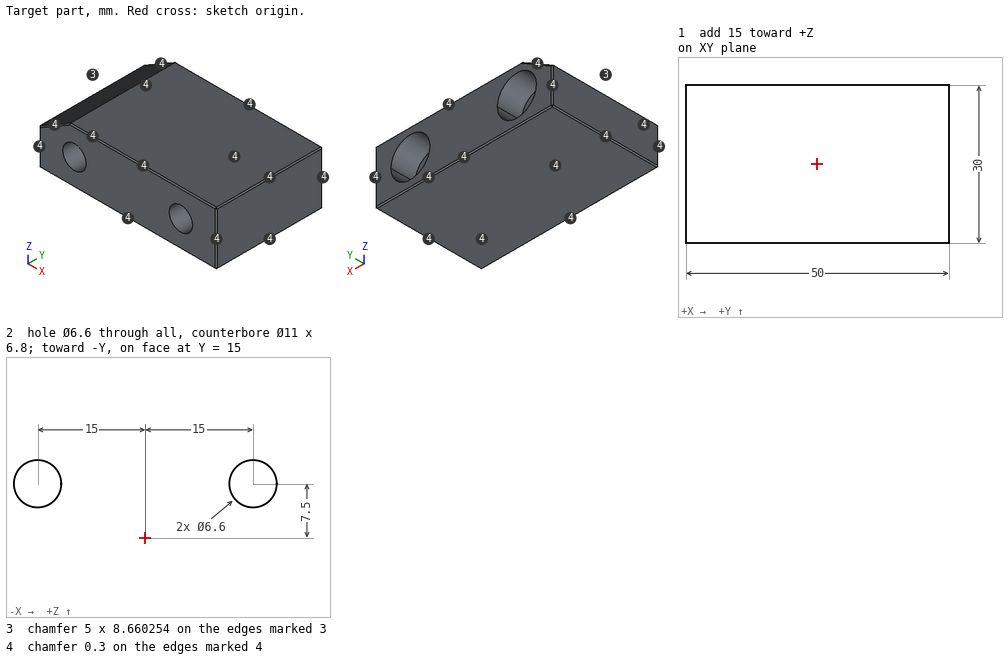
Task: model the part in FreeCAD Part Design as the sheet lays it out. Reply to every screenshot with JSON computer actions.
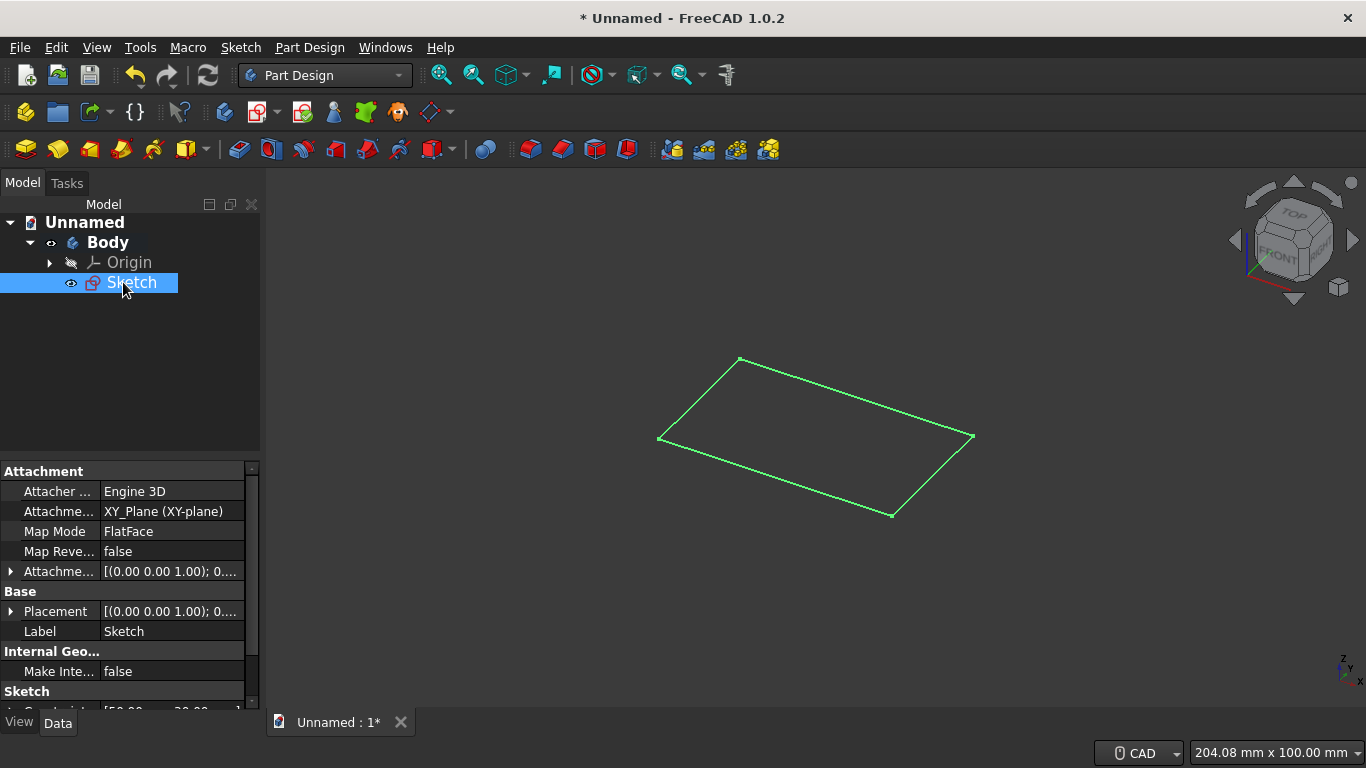
{"action": "left_click", "coordinate": [26, 150]}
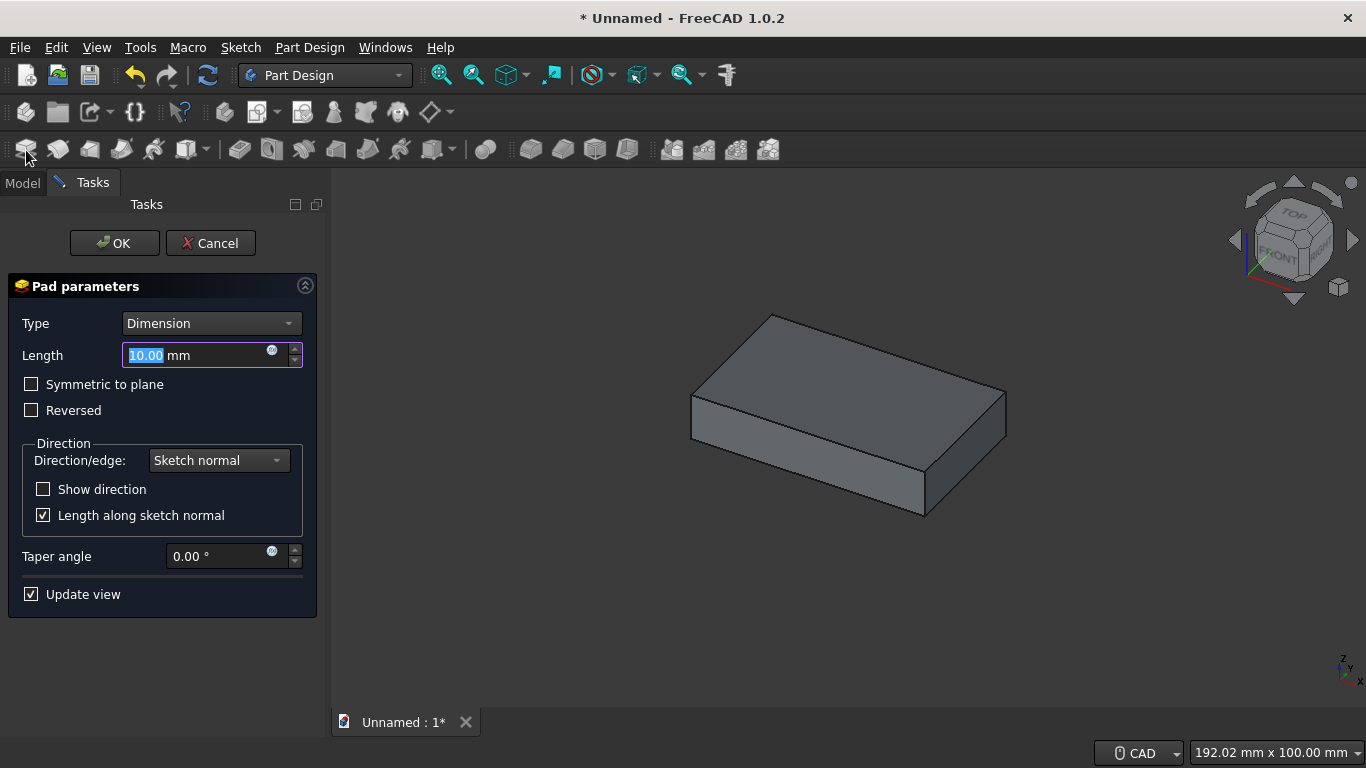
{"action": "type", "text": "15"}
{"action": "key", "text": "Tab"}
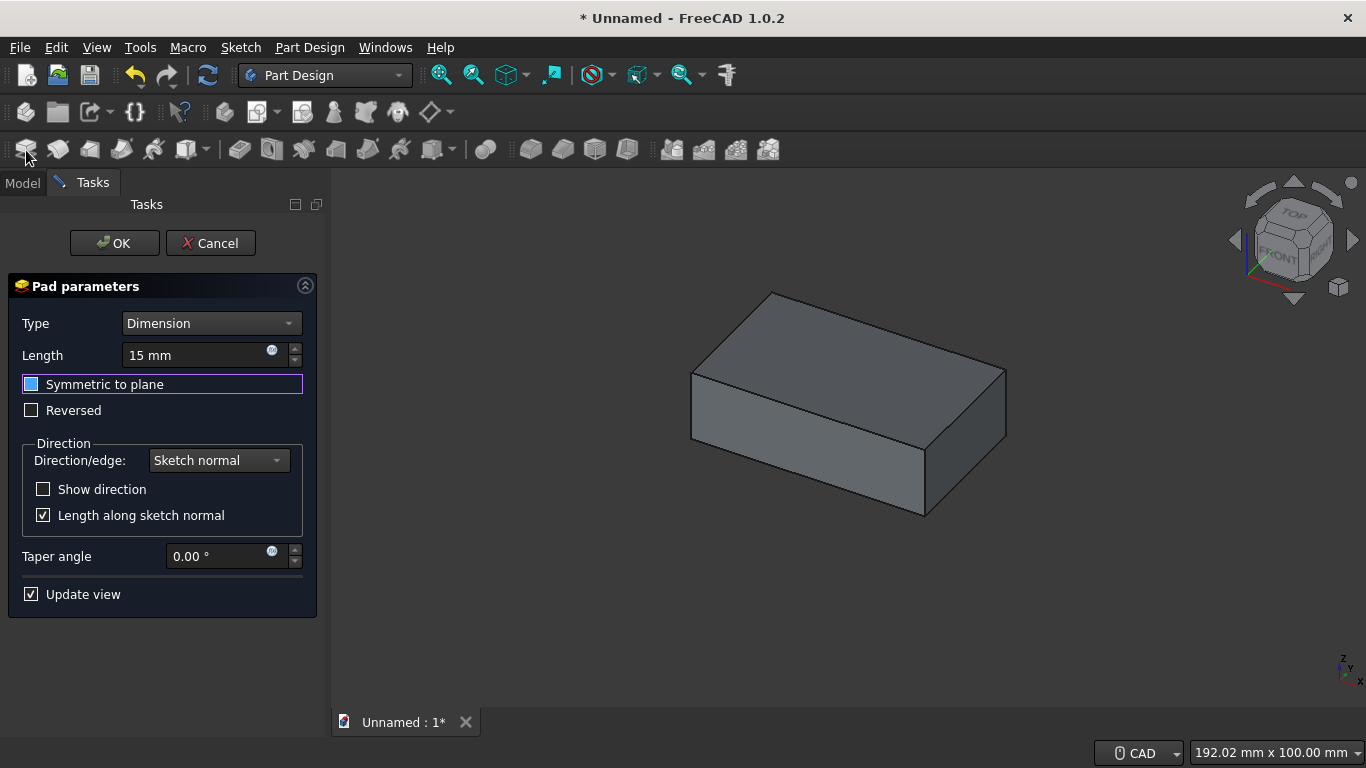
{"action": "left_click", "coordinate": [115, 243]}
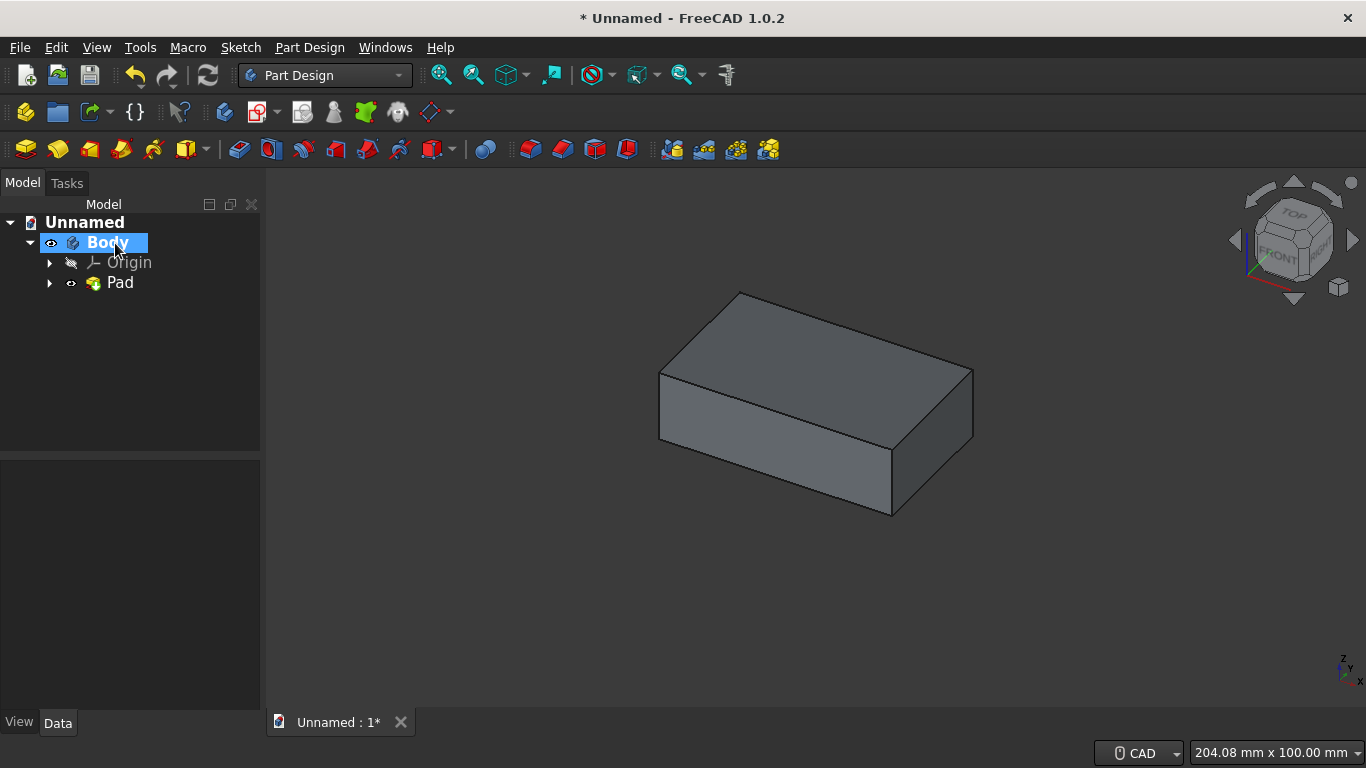
{"action": "left_click", "coordinate": [442, 76]}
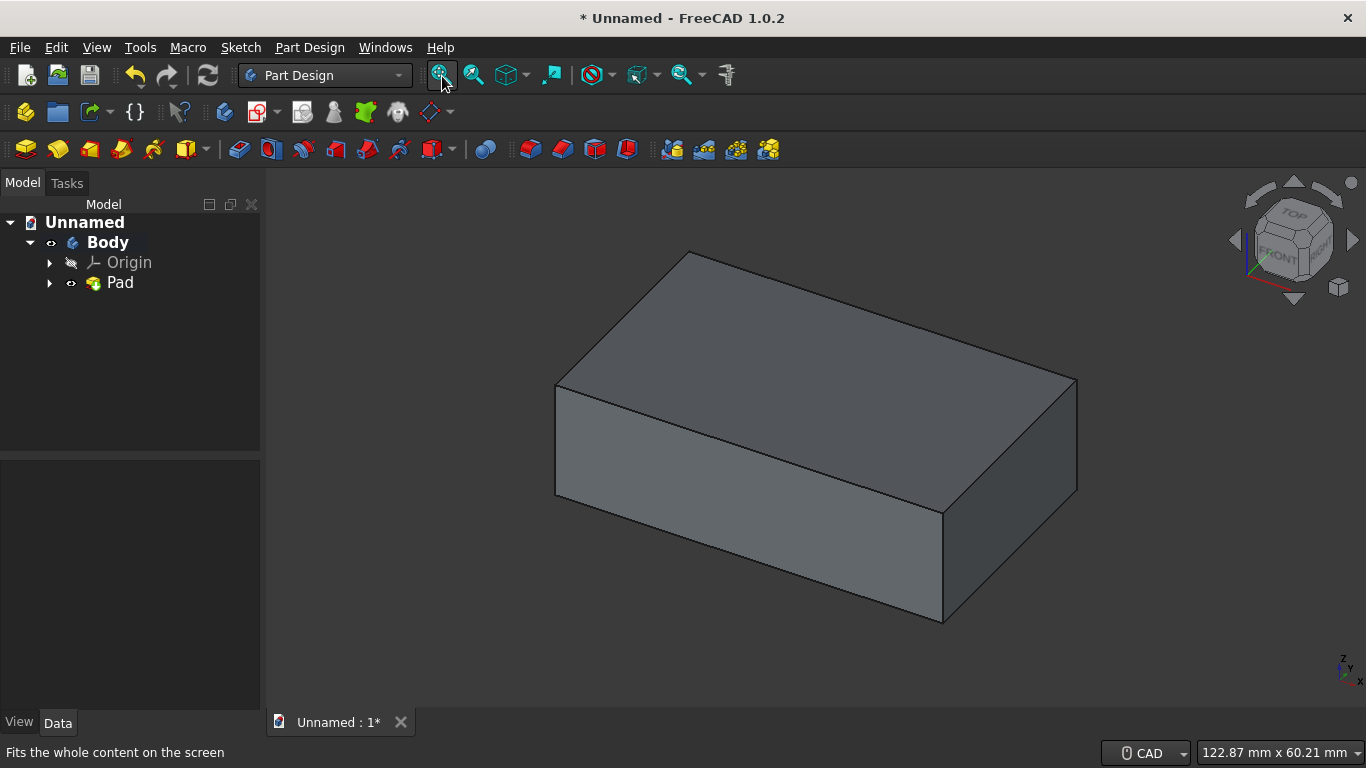
{"action": "key", "text": "4"}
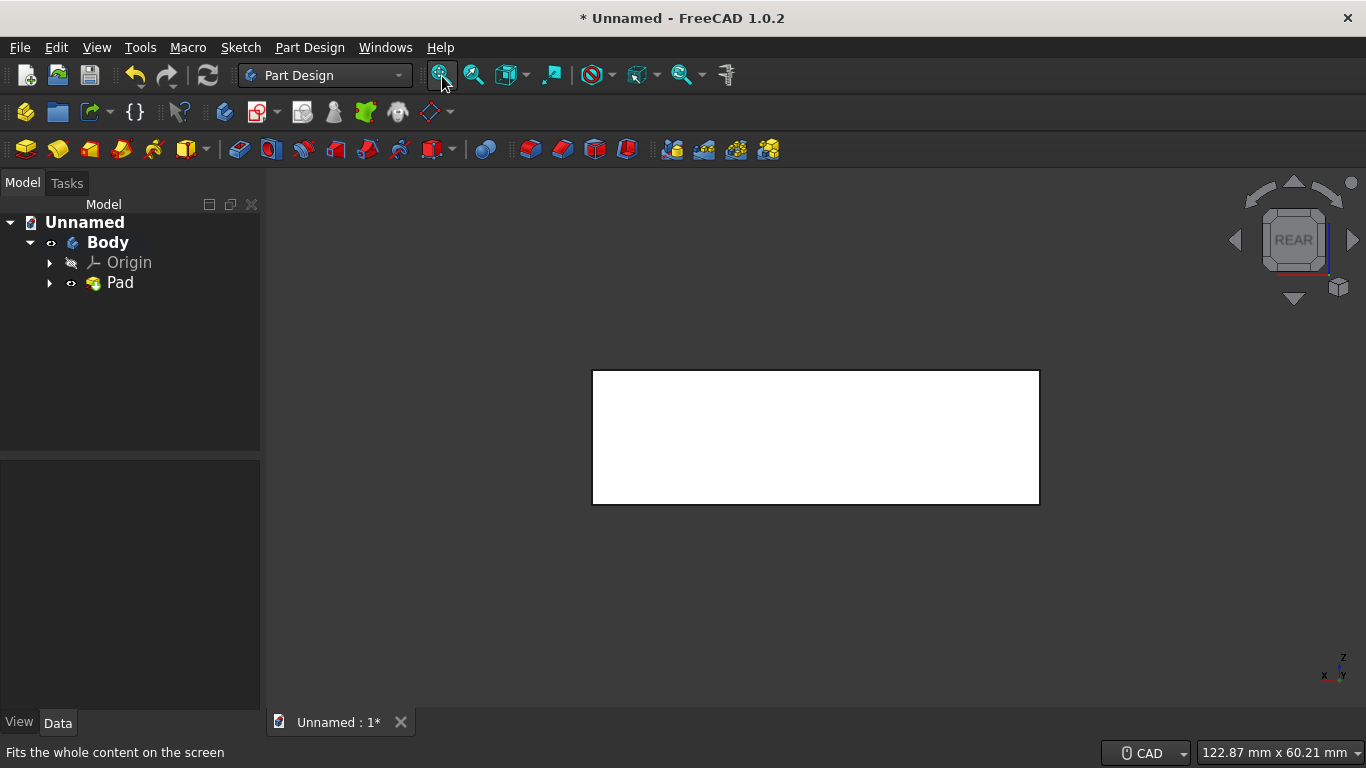
{"action": "left_click", "coordinate": [442, 76]}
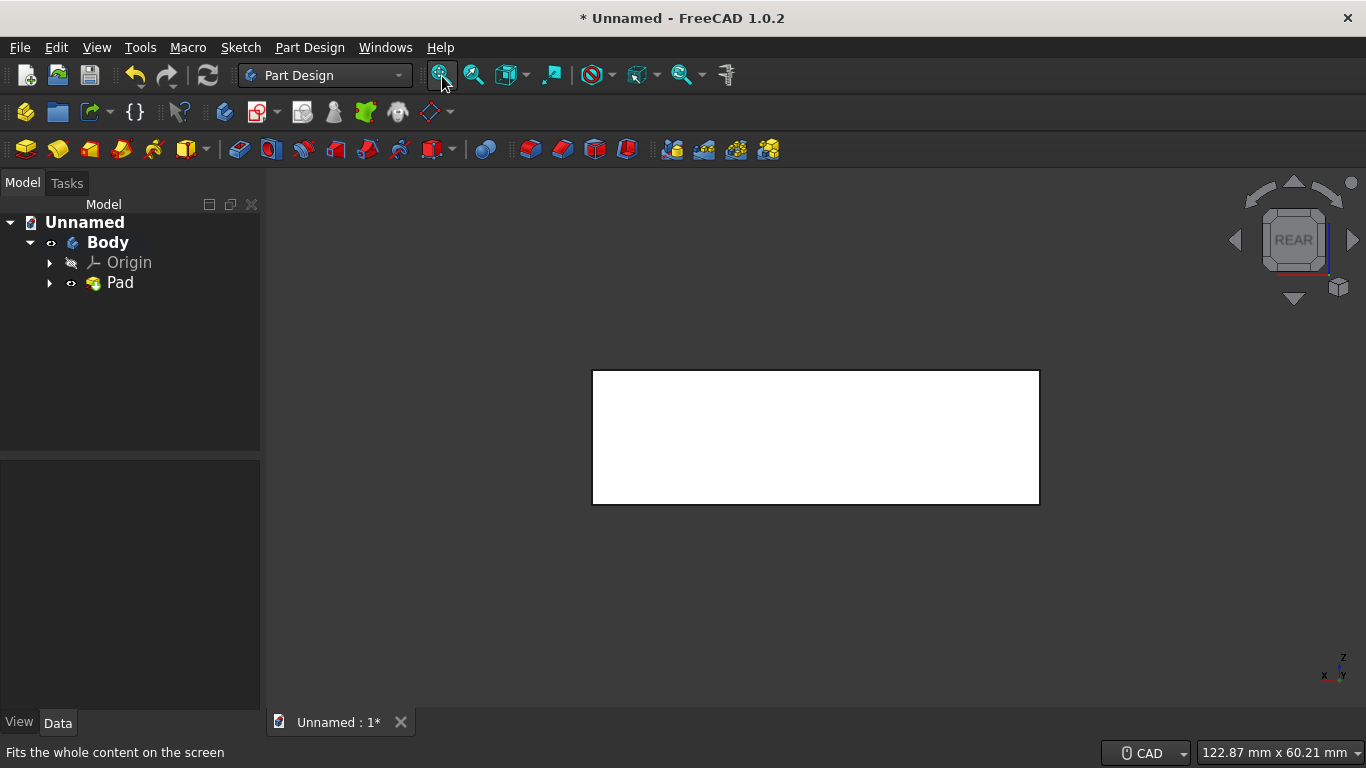
{"action": "left_click", "coordinate": [688, 437]}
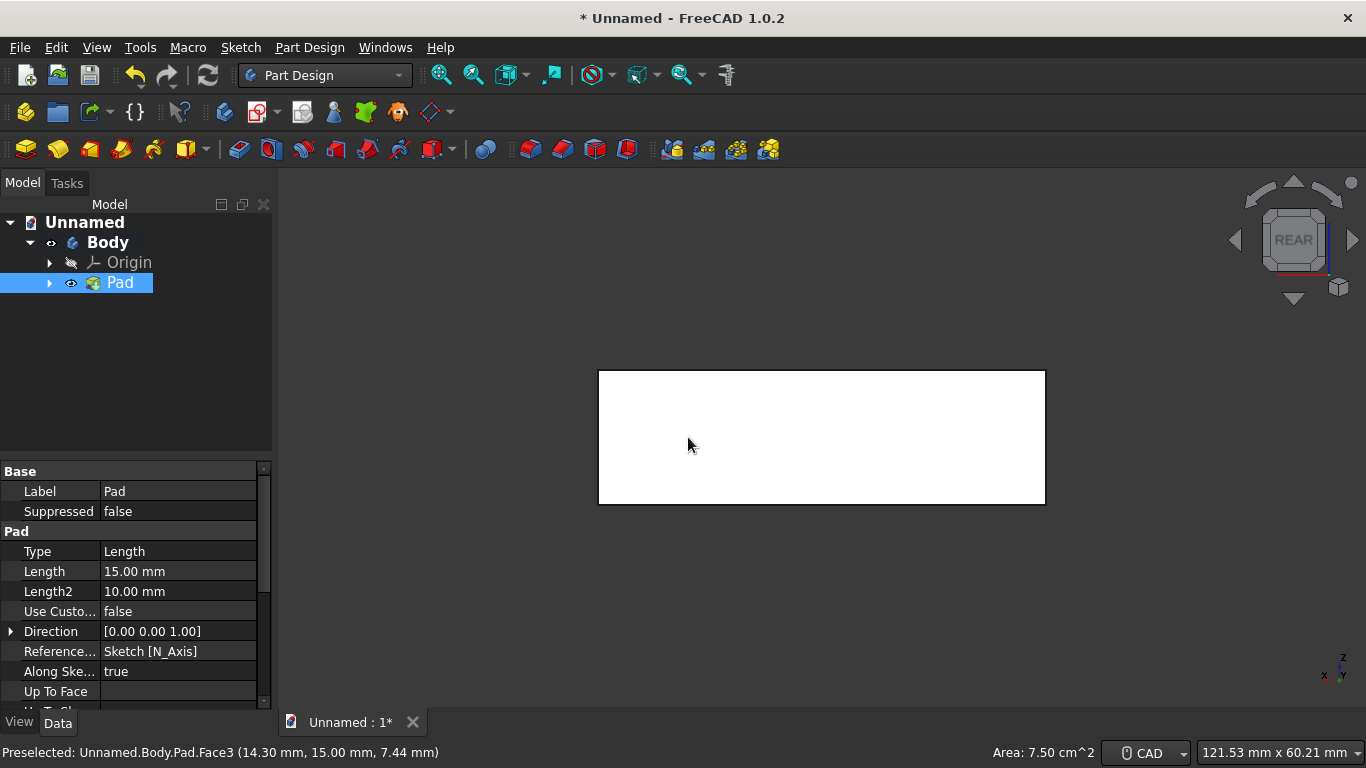
{"action": "left_click", "coordinate": [258, 112]}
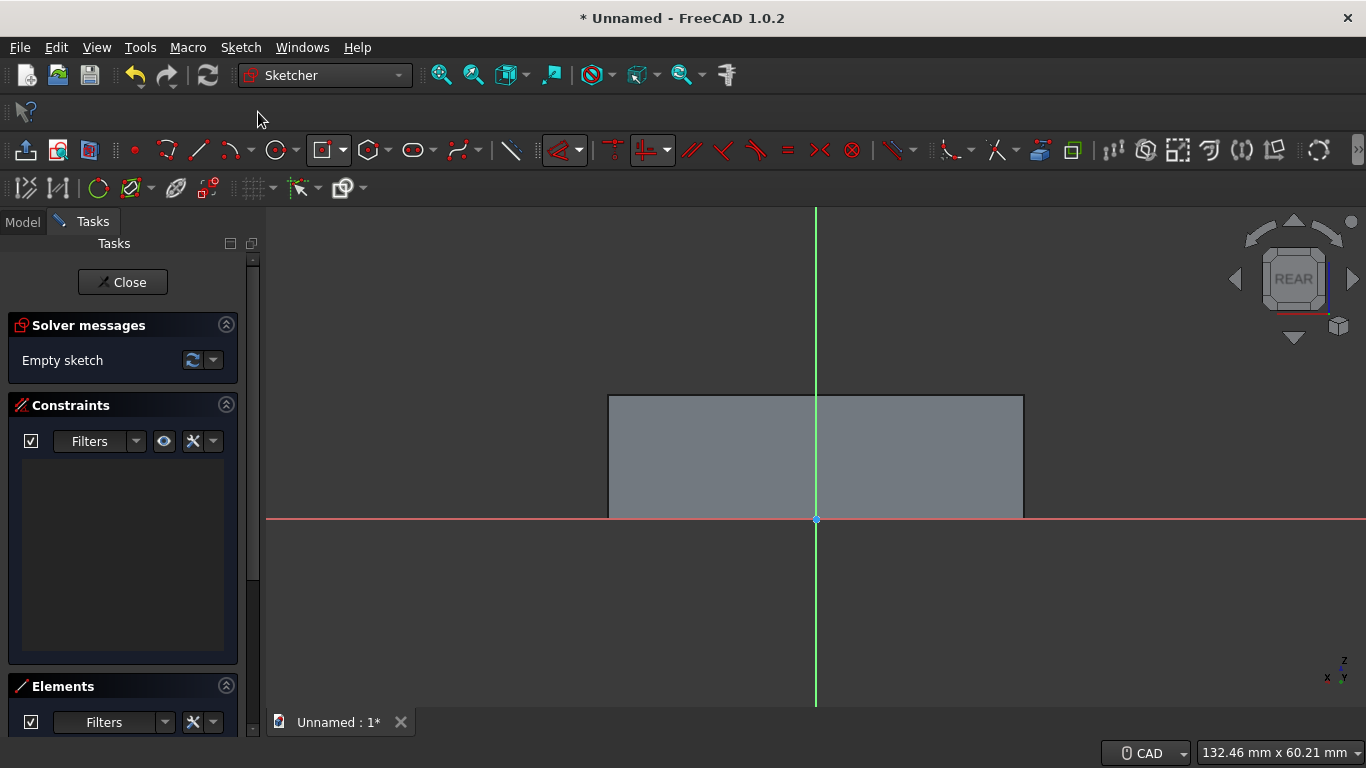
{"action": "scroll", "coordinate": [872, 489], "scroll_direction": "up", "scroll_amount": 4}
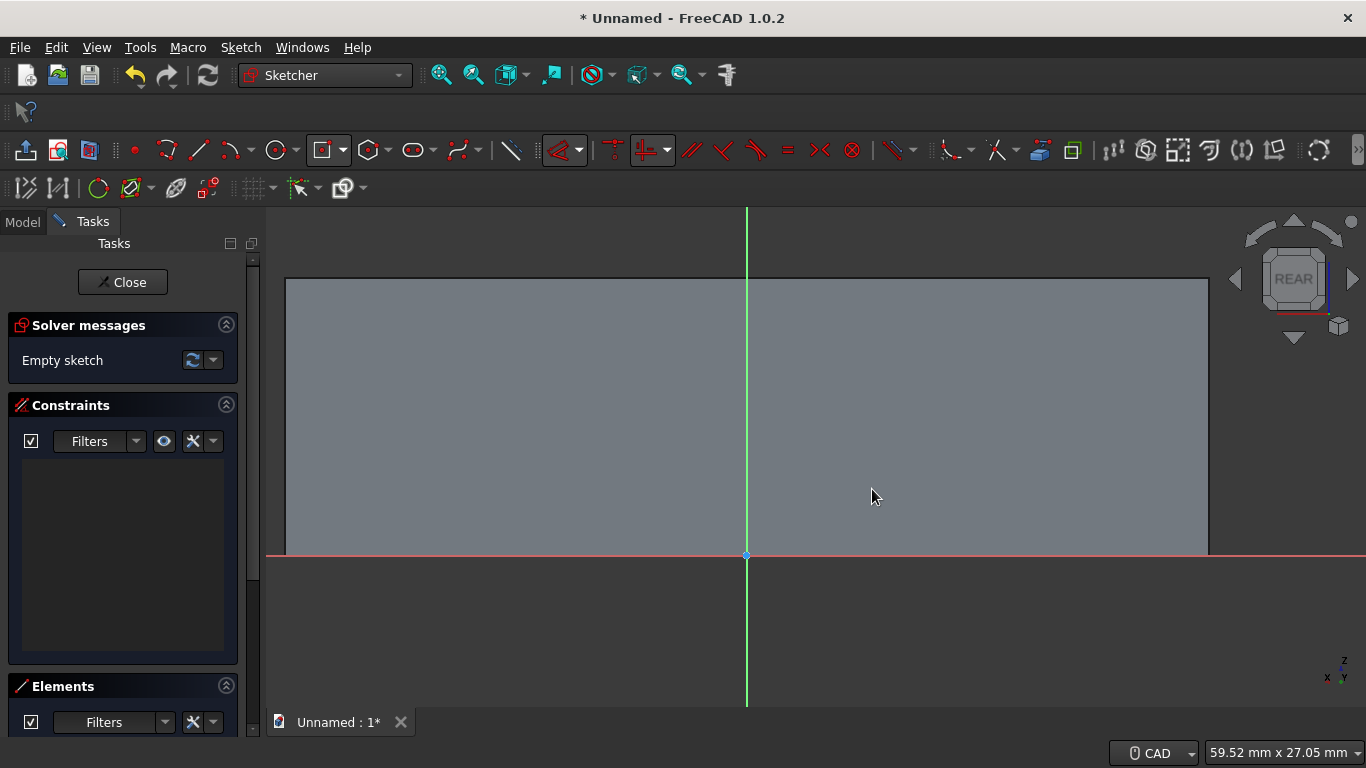
{"action": "left_click", "coordinate": [276, 150]}